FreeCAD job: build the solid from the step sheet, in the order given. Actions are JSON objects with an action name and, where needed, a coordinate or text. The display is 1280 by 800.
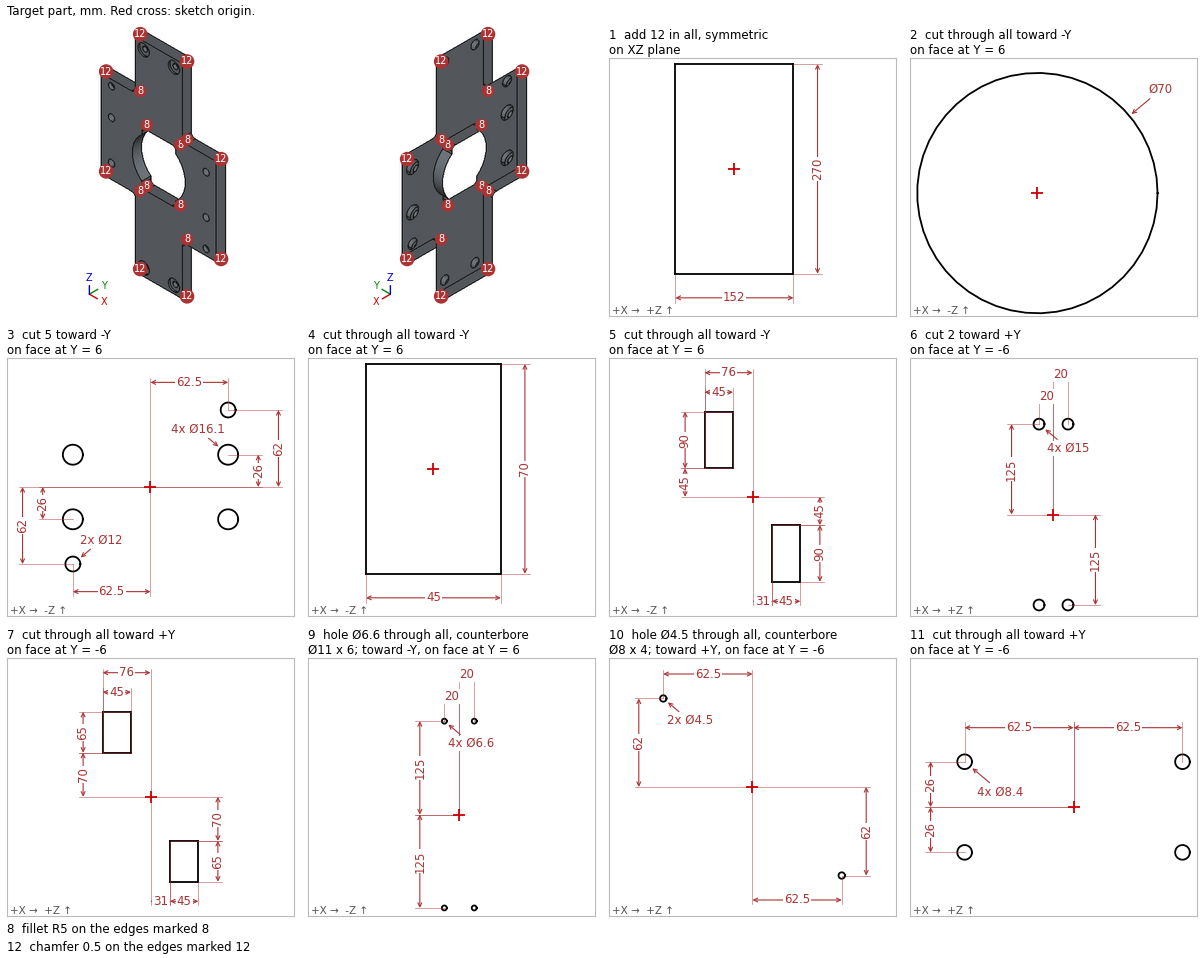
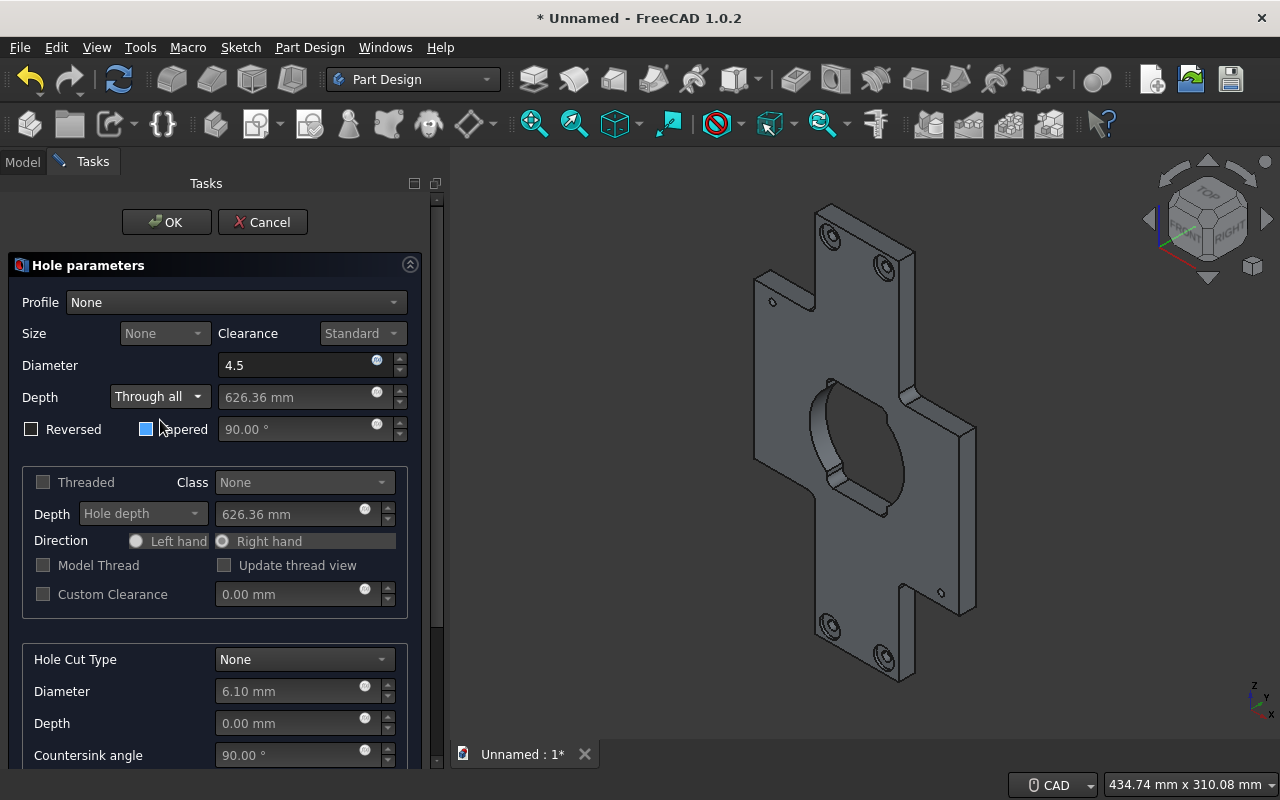
{"action": "left_click", "coordinate": [306, 660]}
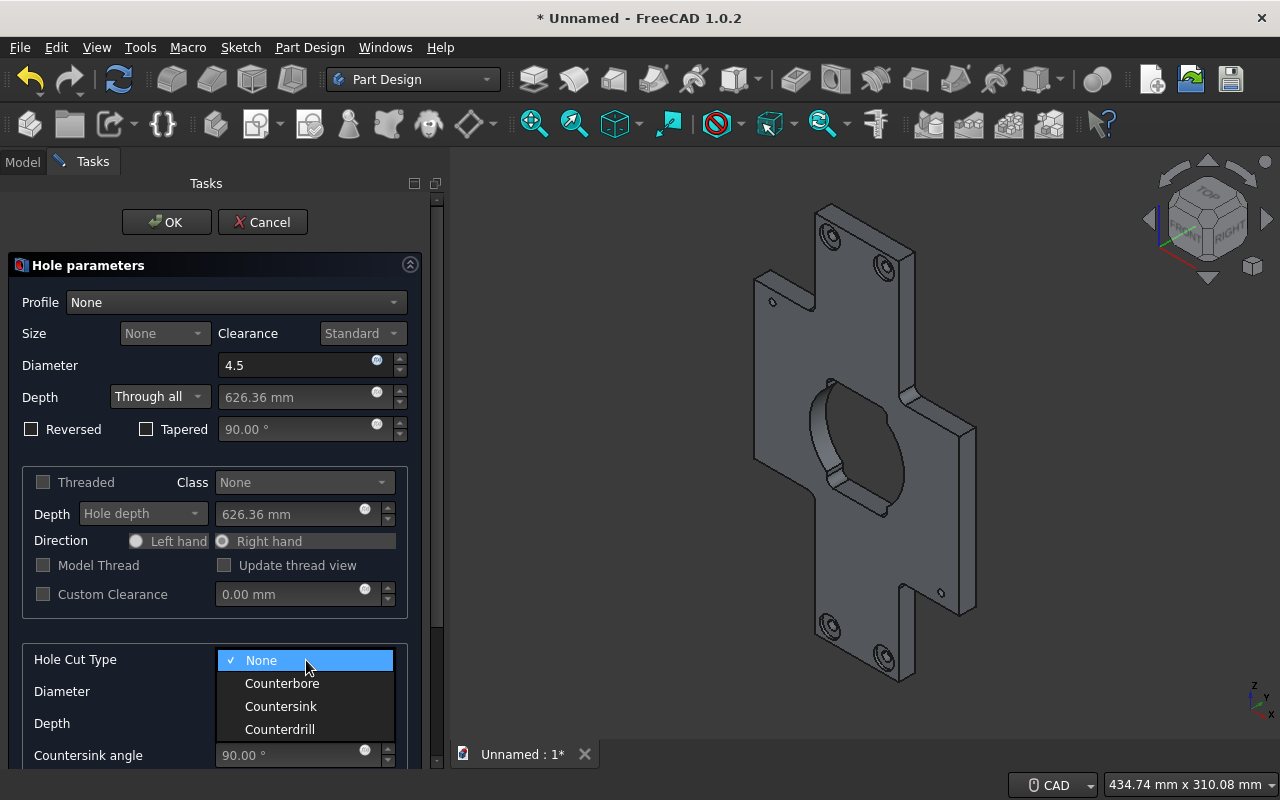
{"action": "left_click", "coordinate": [304, 684]}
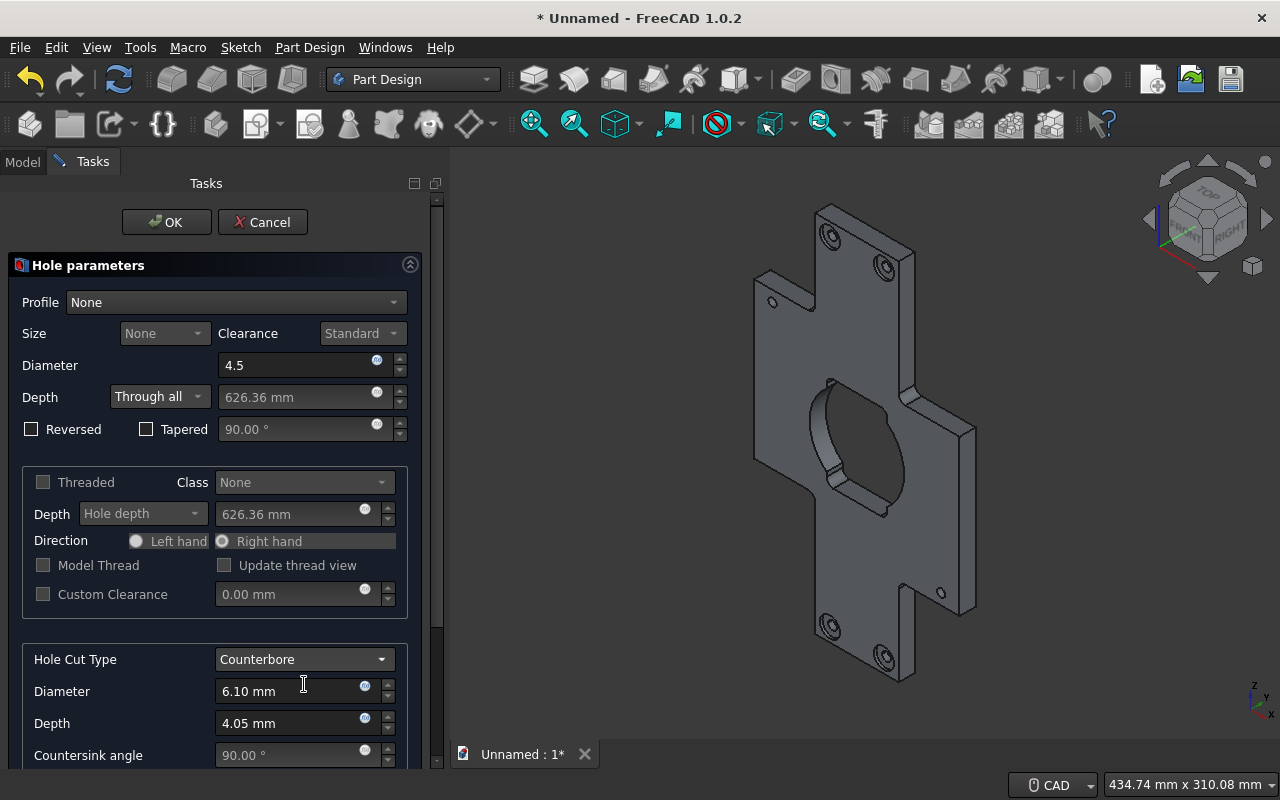
{"action": "triple_click", "coordinate": [298, 691]}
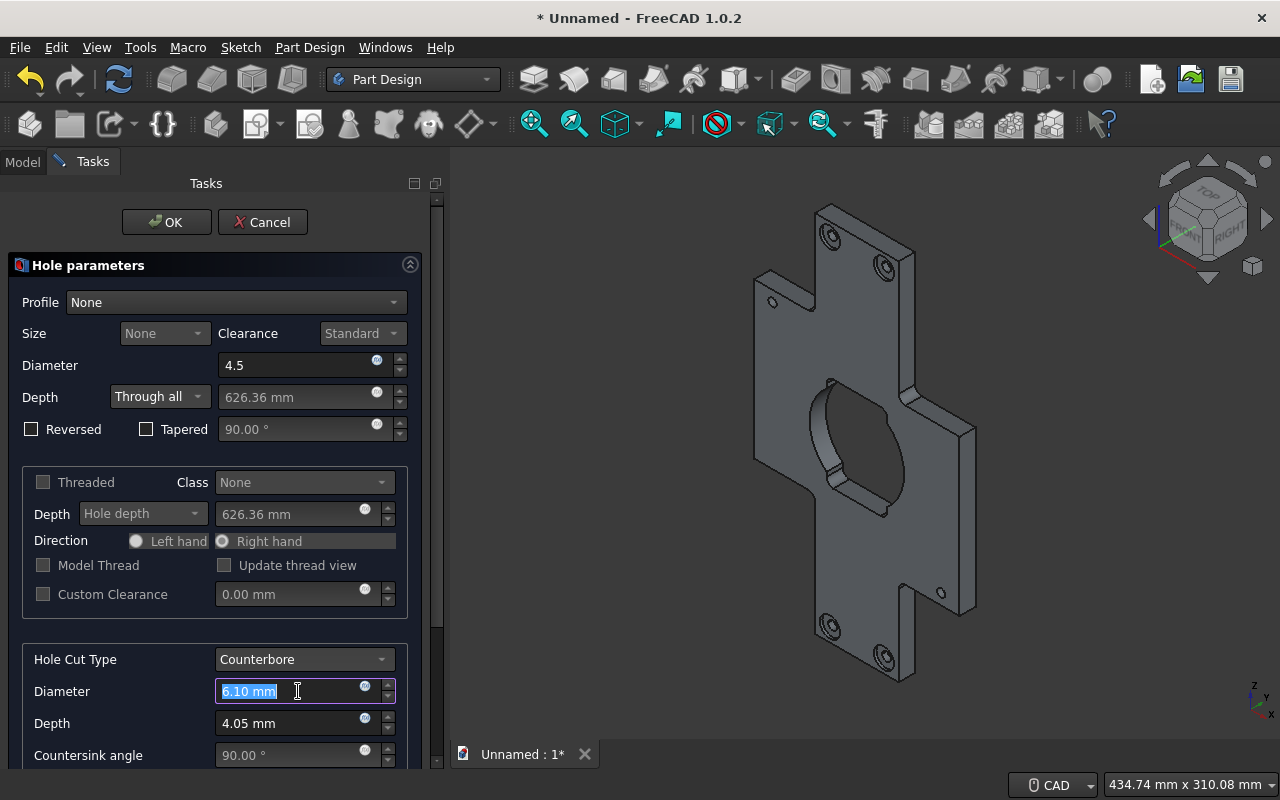
{"action": "type", "text": "8"}
{"action": "key", "text": "Tab"}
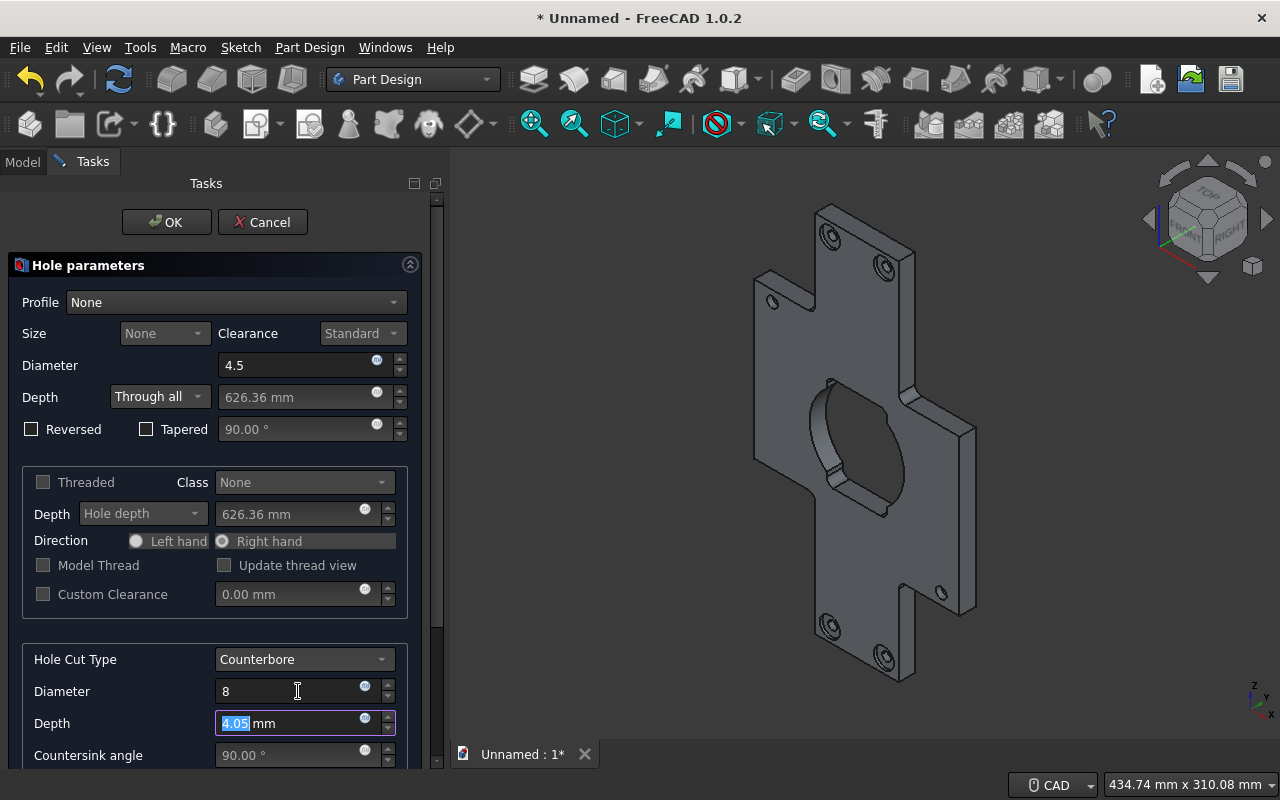
{"action": "type", "text": "4"}
{"action": "key", "text": "Tab"}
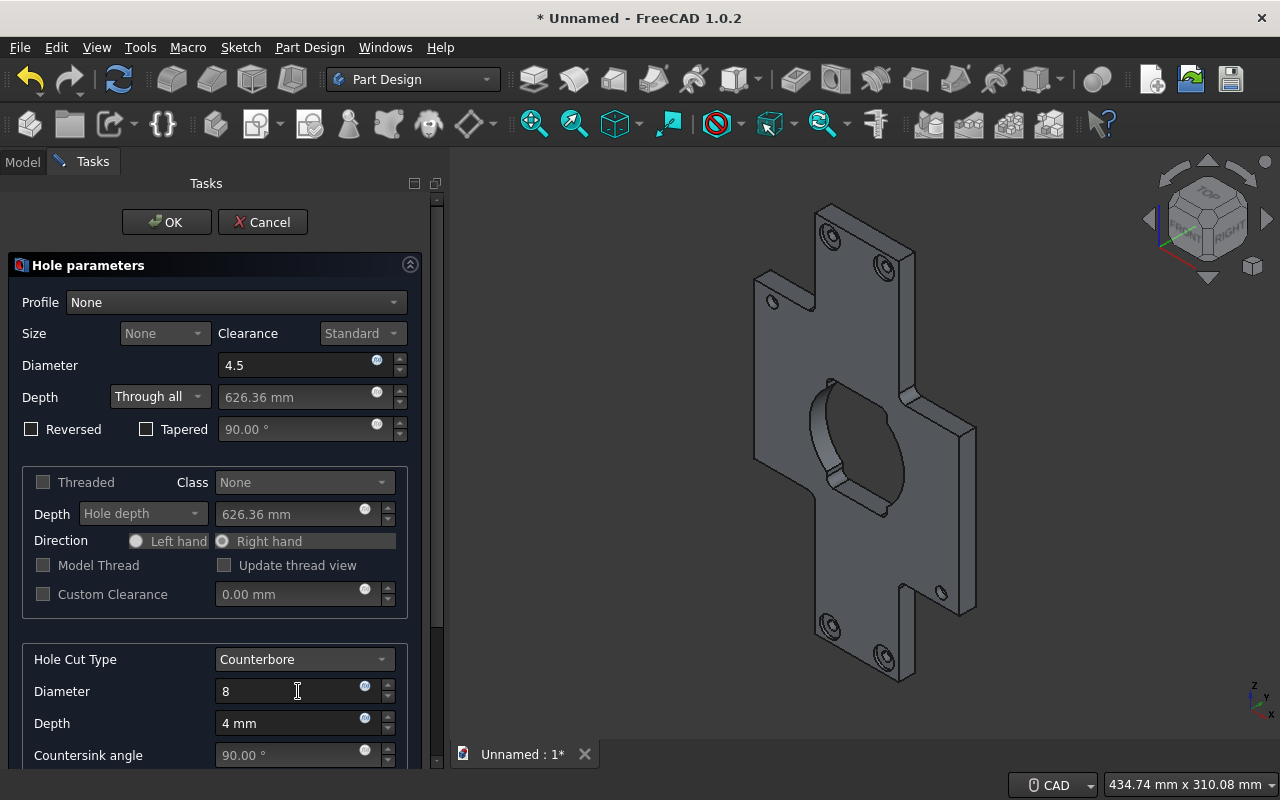
{"action": "left_click", "coordinate": [167, 222]}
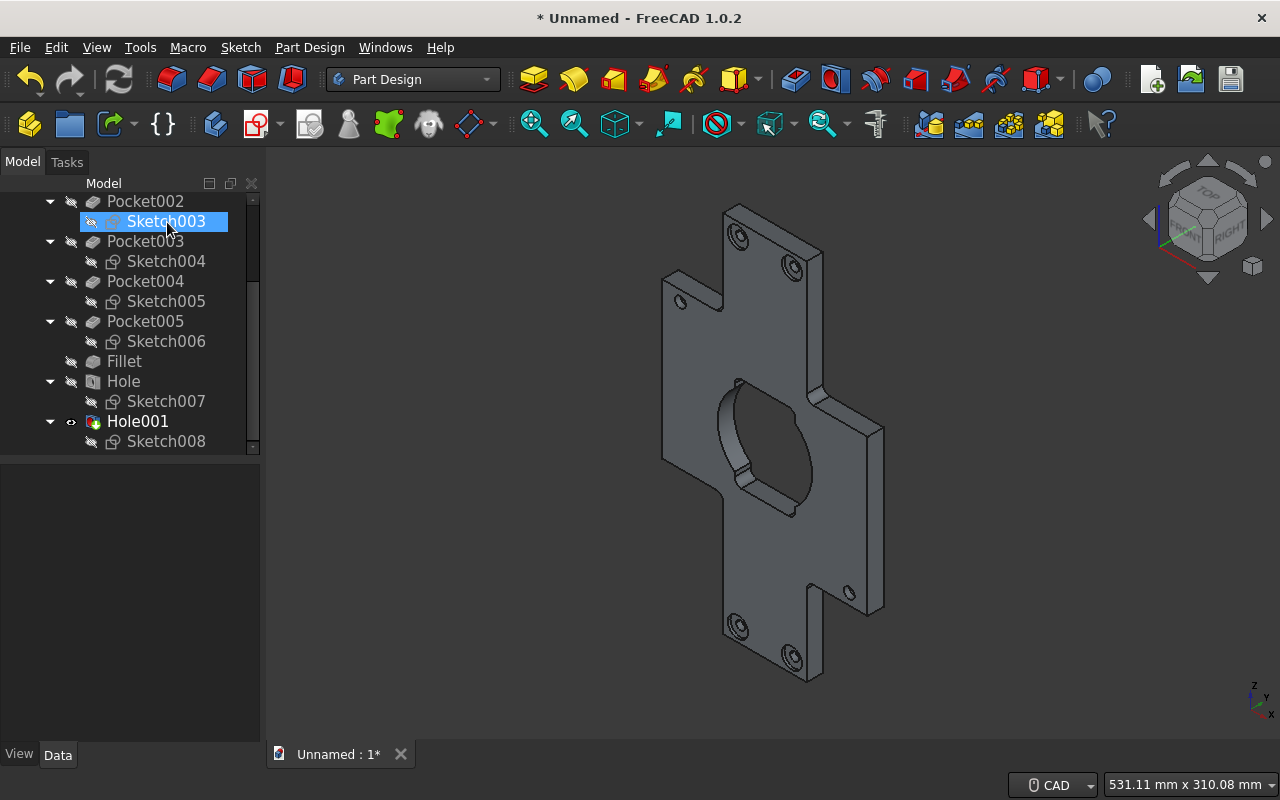
{"action": "left_click", "coordinate": [765, 326]}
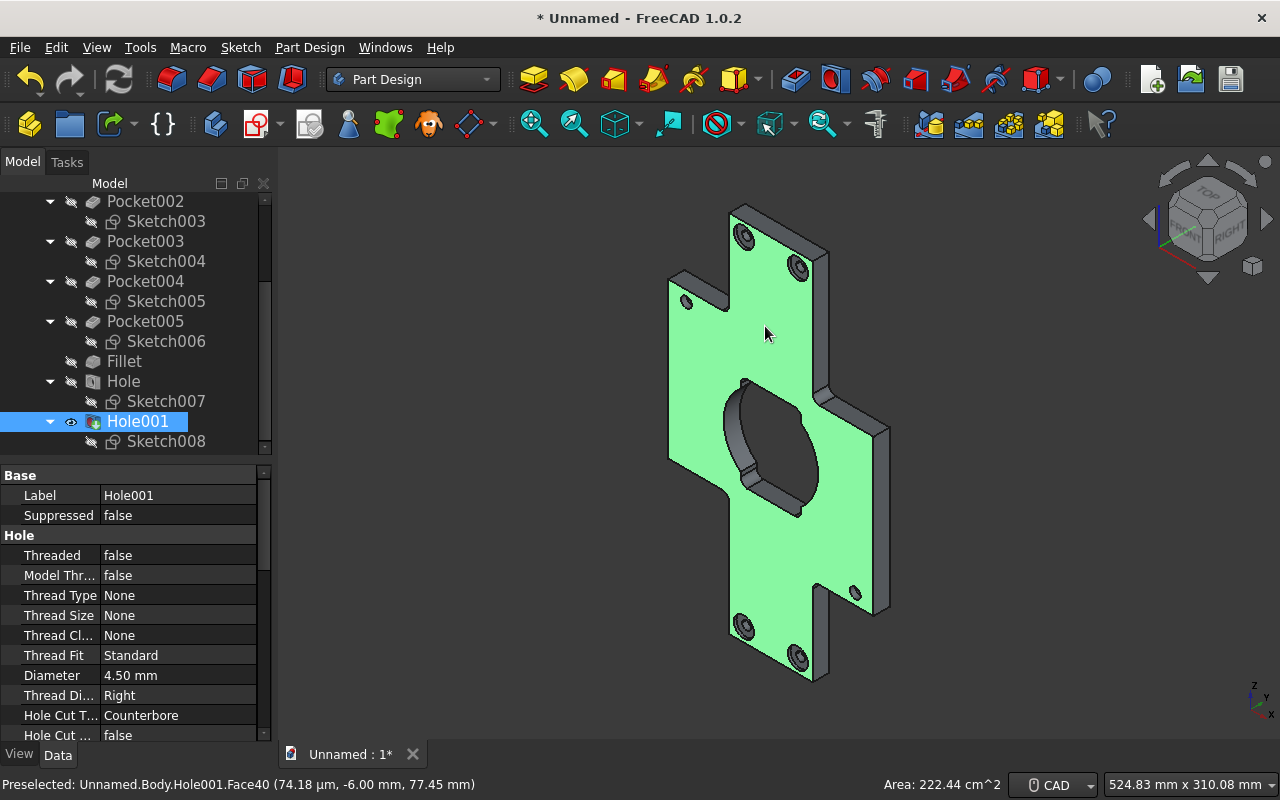
{"action": "left_click", "coordinate": [256, 124]}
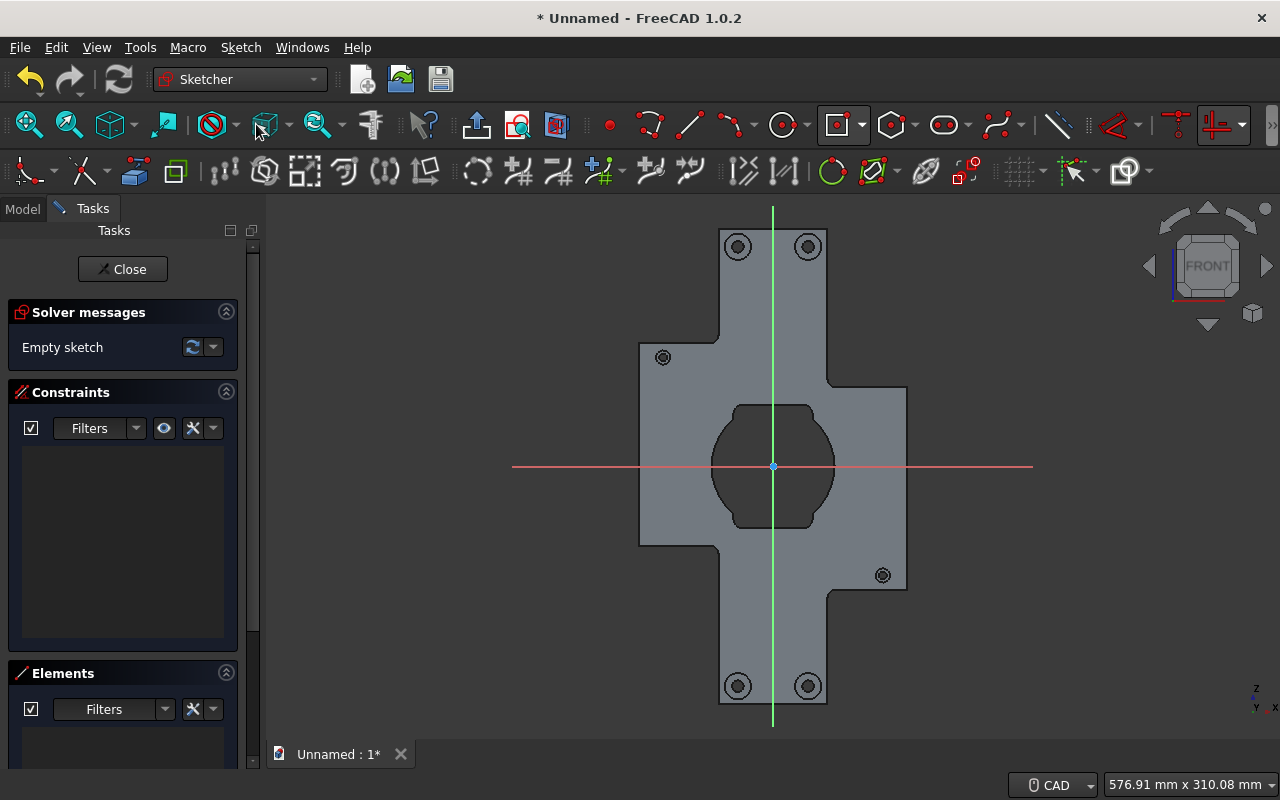
{"action": "scroll", "coordinate": [813, 466], "scroll_direction": "up", "scroll_amount": 5}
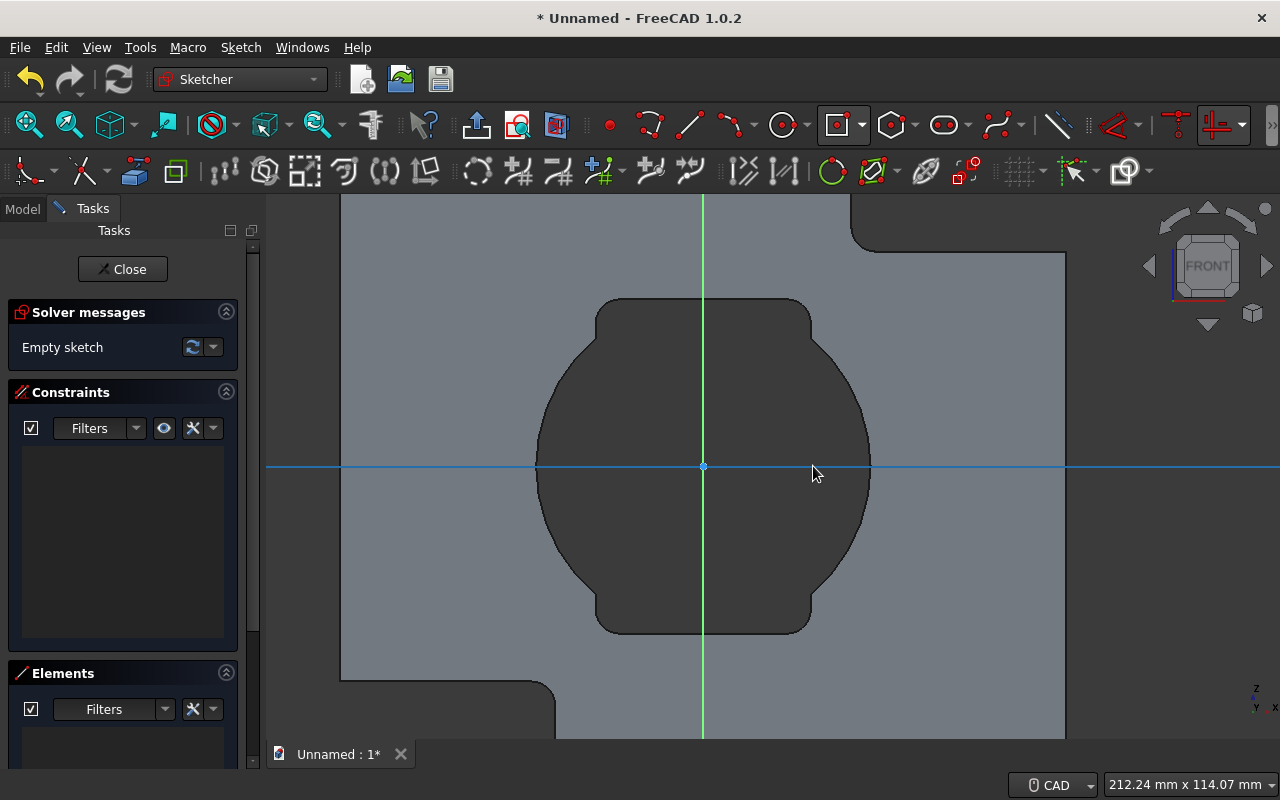
{"action": "key", "text": "g c"}